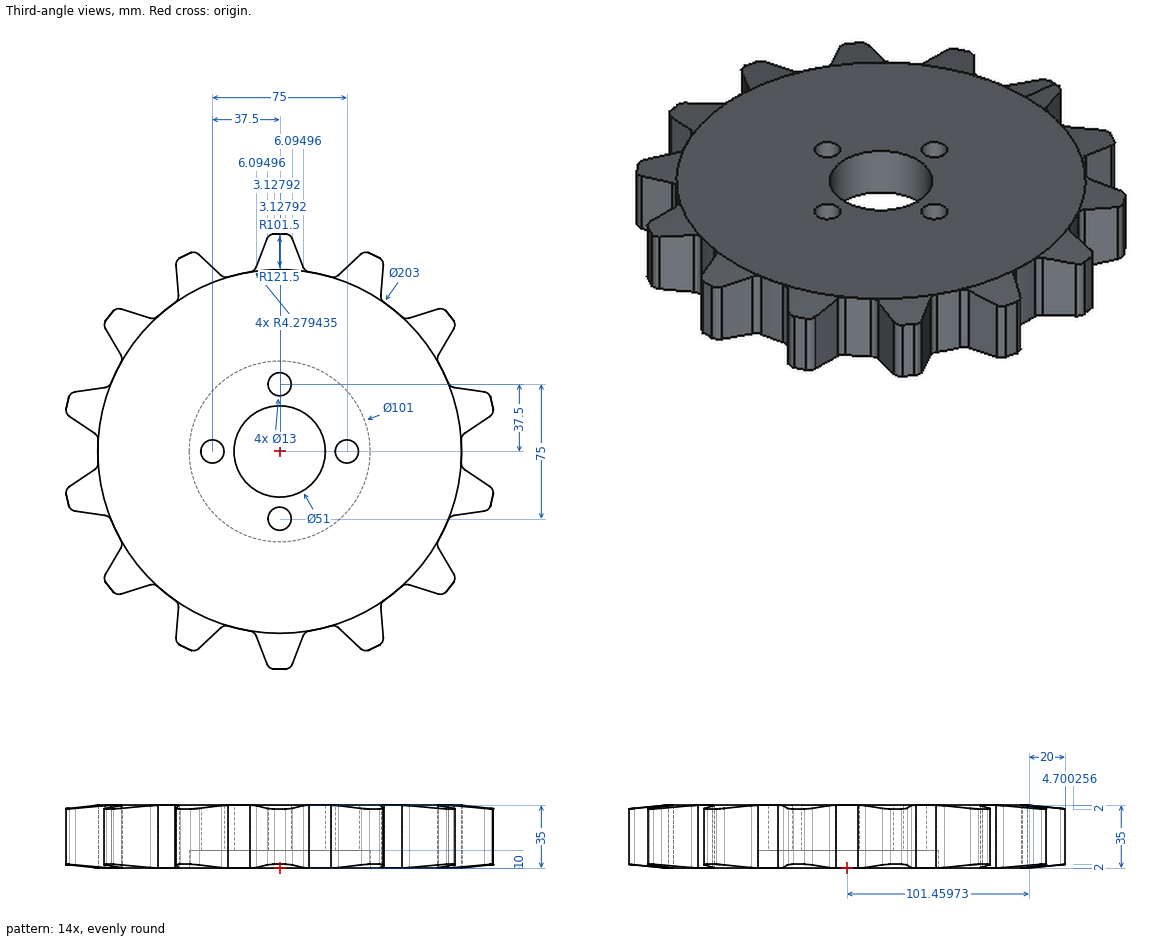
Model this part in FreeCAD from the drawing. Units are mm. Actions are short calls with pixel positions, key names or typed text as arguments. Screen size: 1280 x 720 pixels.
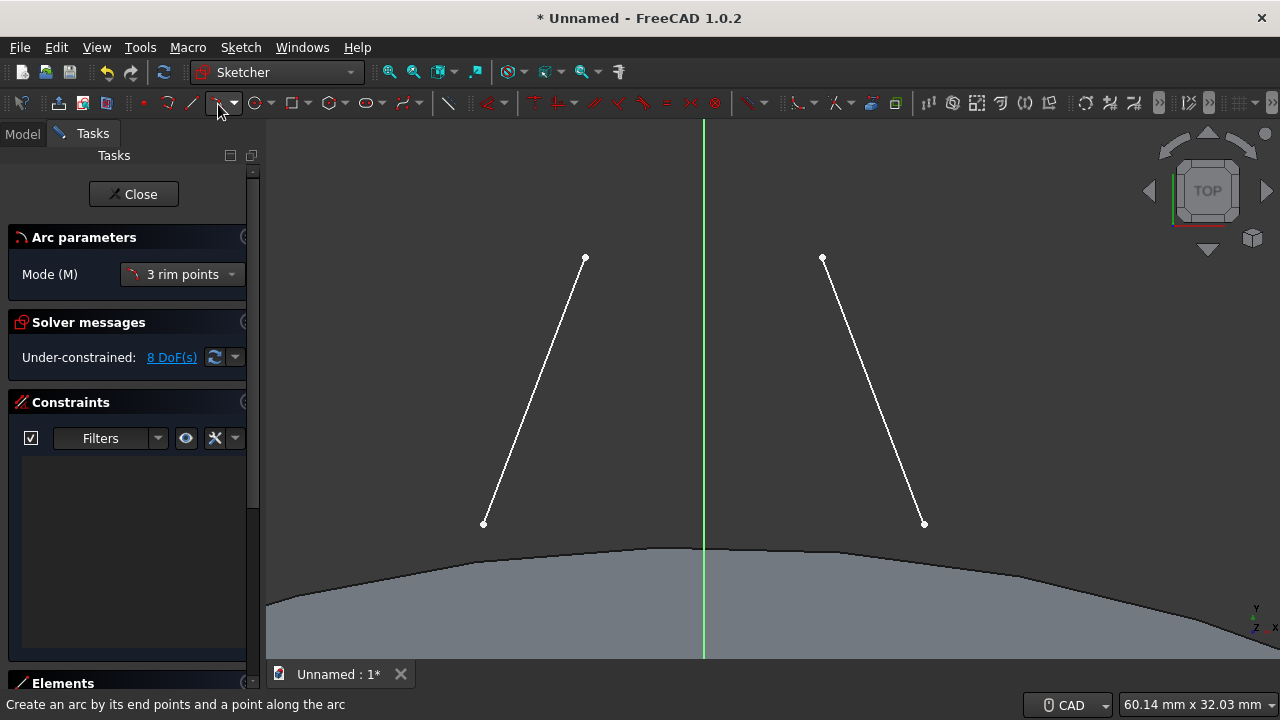
click(483, 525)
click(427, 570)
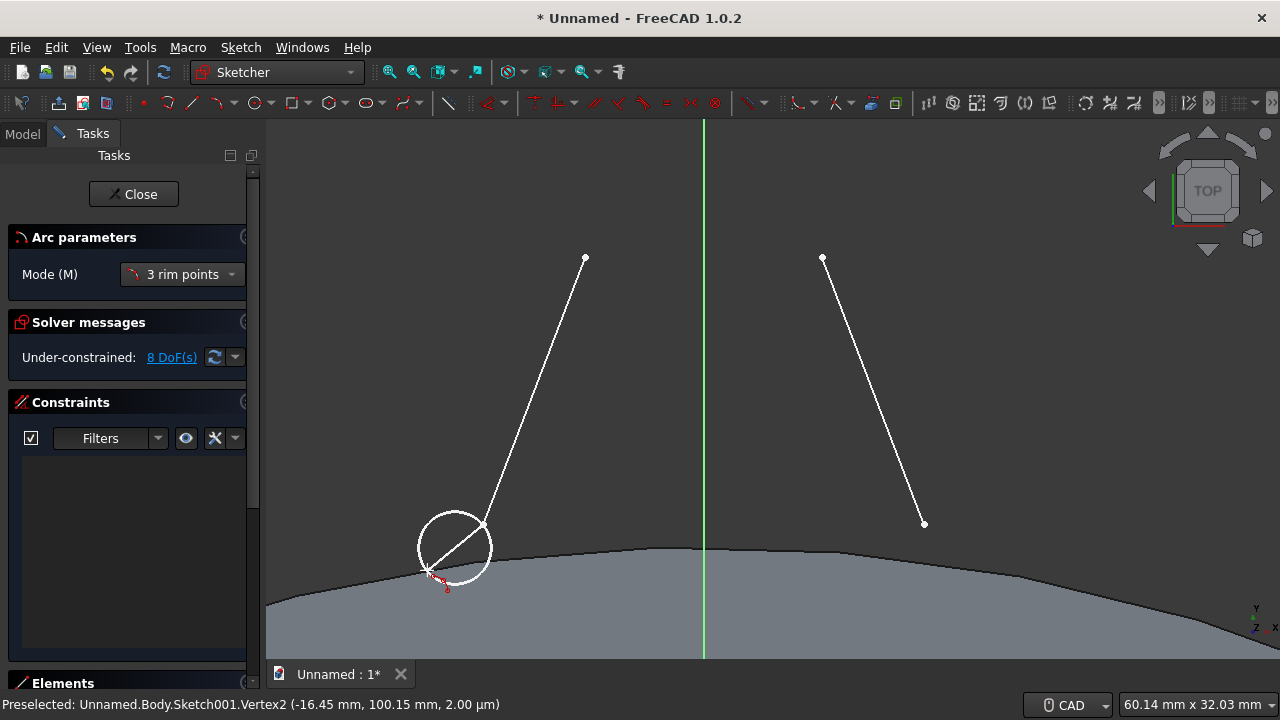
scroll(461, 554, up, 3)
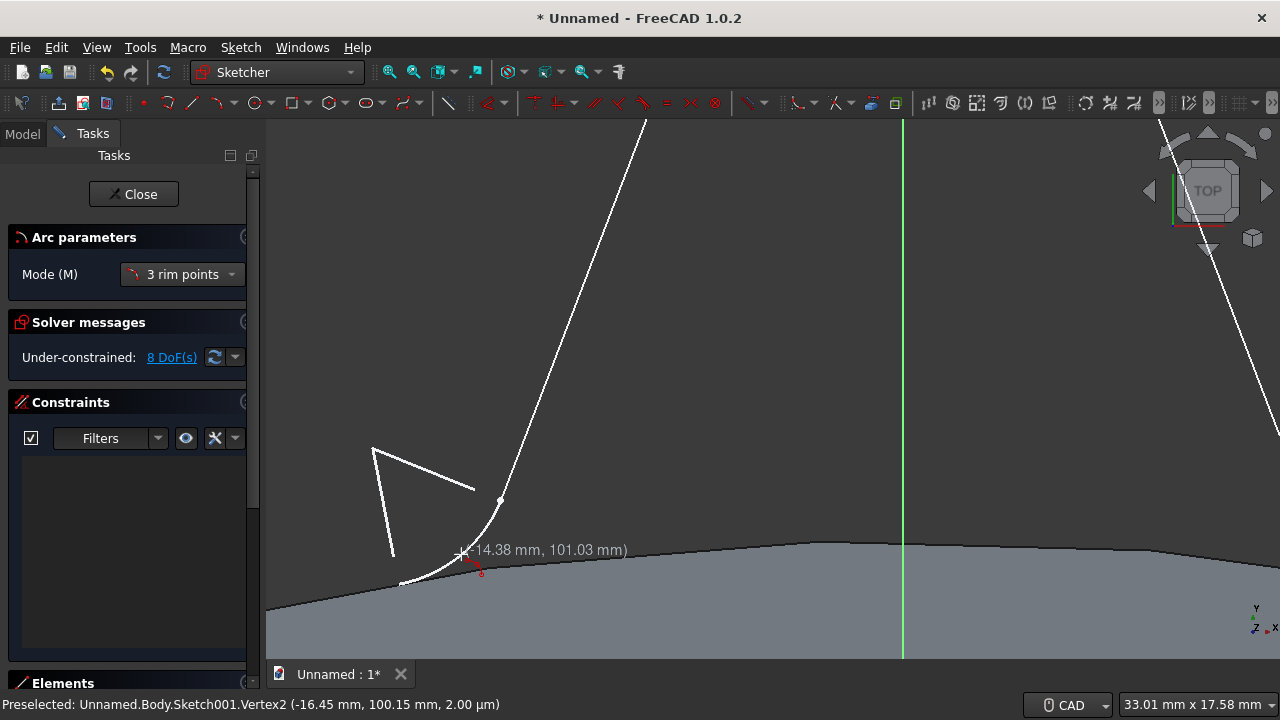
click(460, 554)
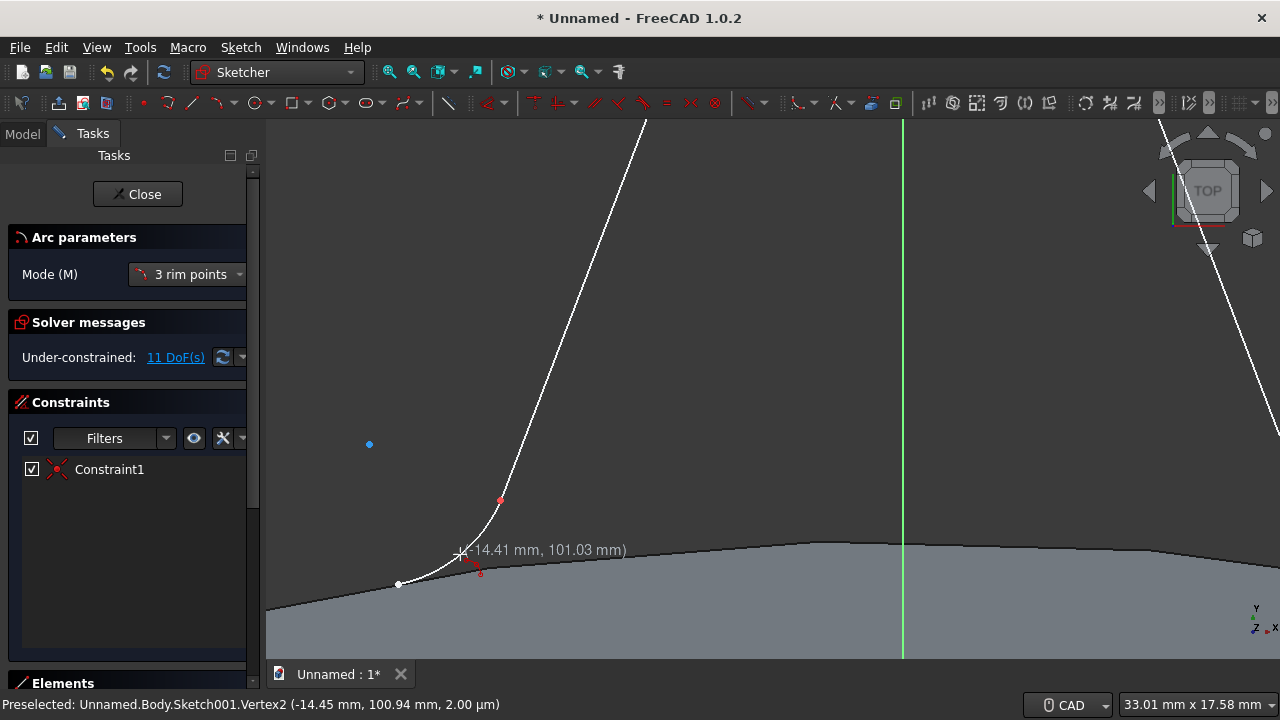
click(399, 584)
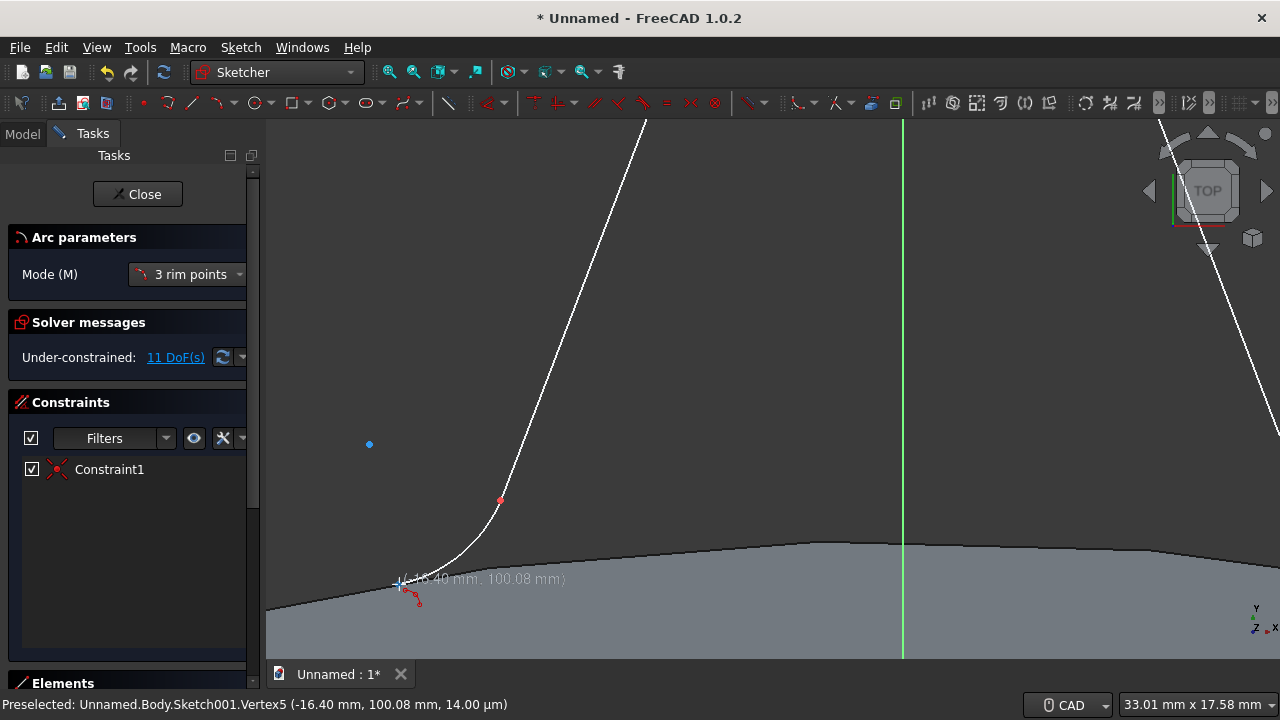
scroll(463, 553, down, 3)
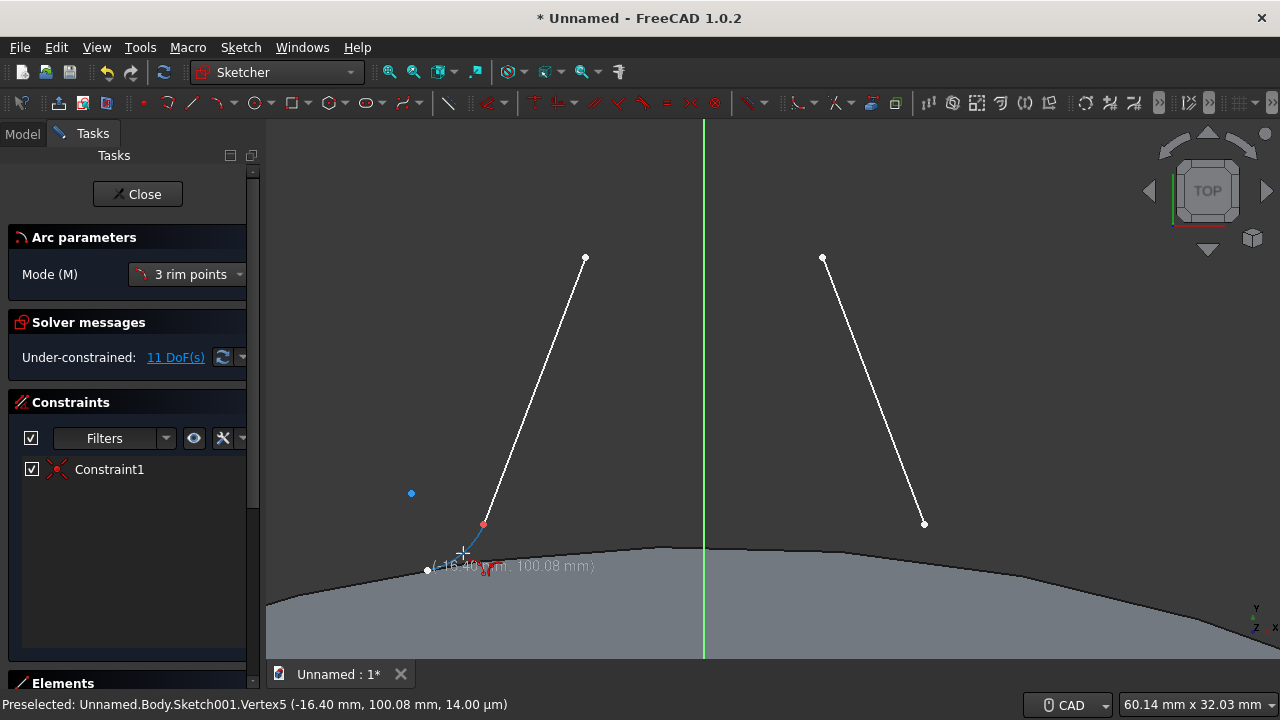
click(981, 569)
click(760, 547)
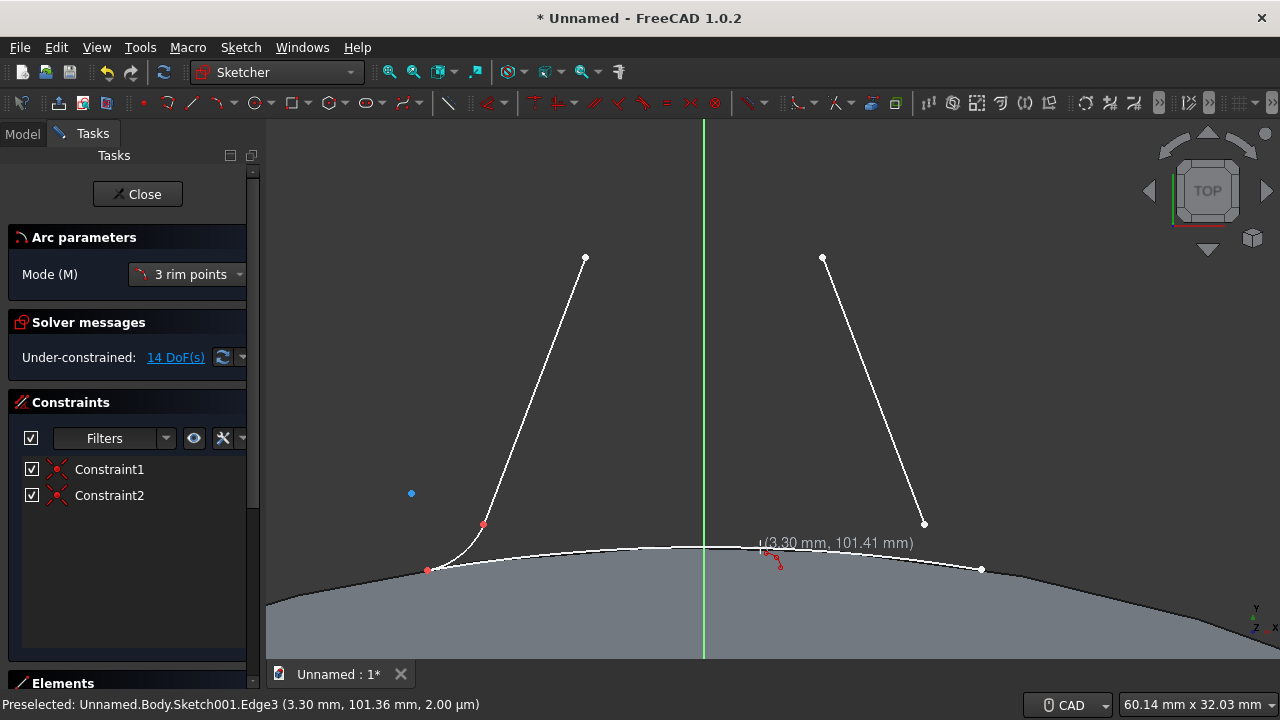
click(981, 570)
click(925, 525)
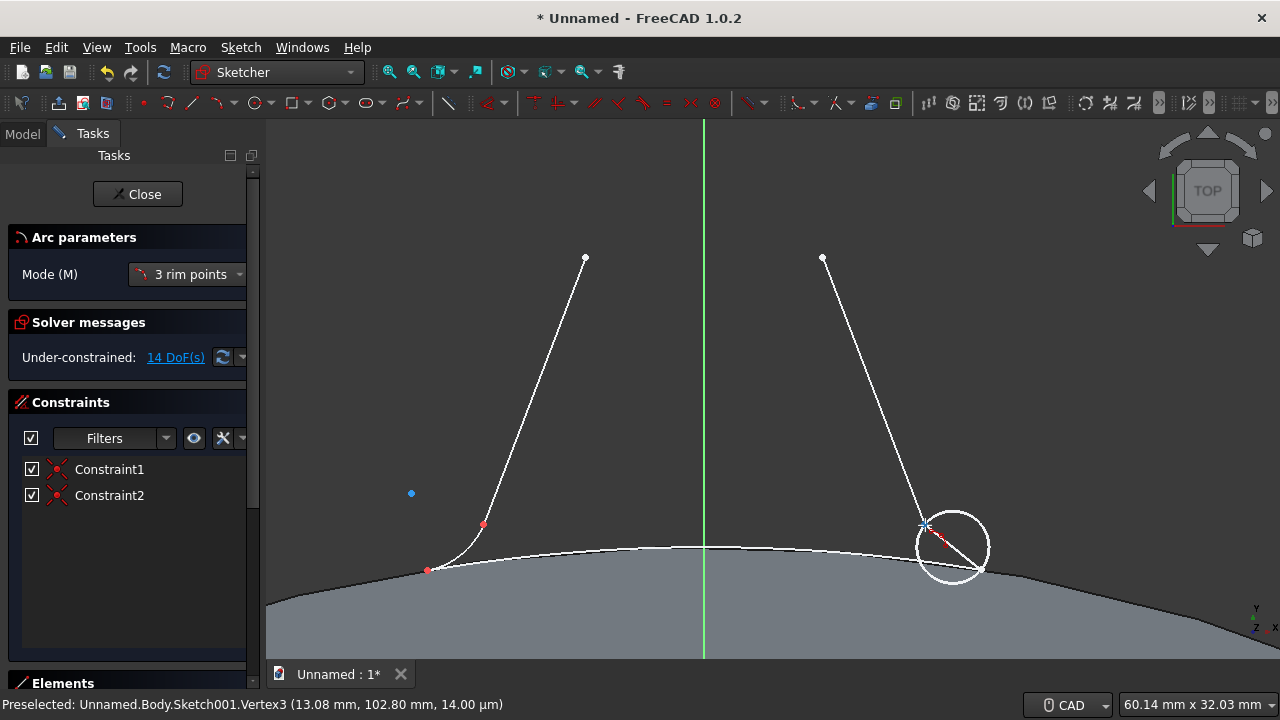
scroll(947, 554, up, 3)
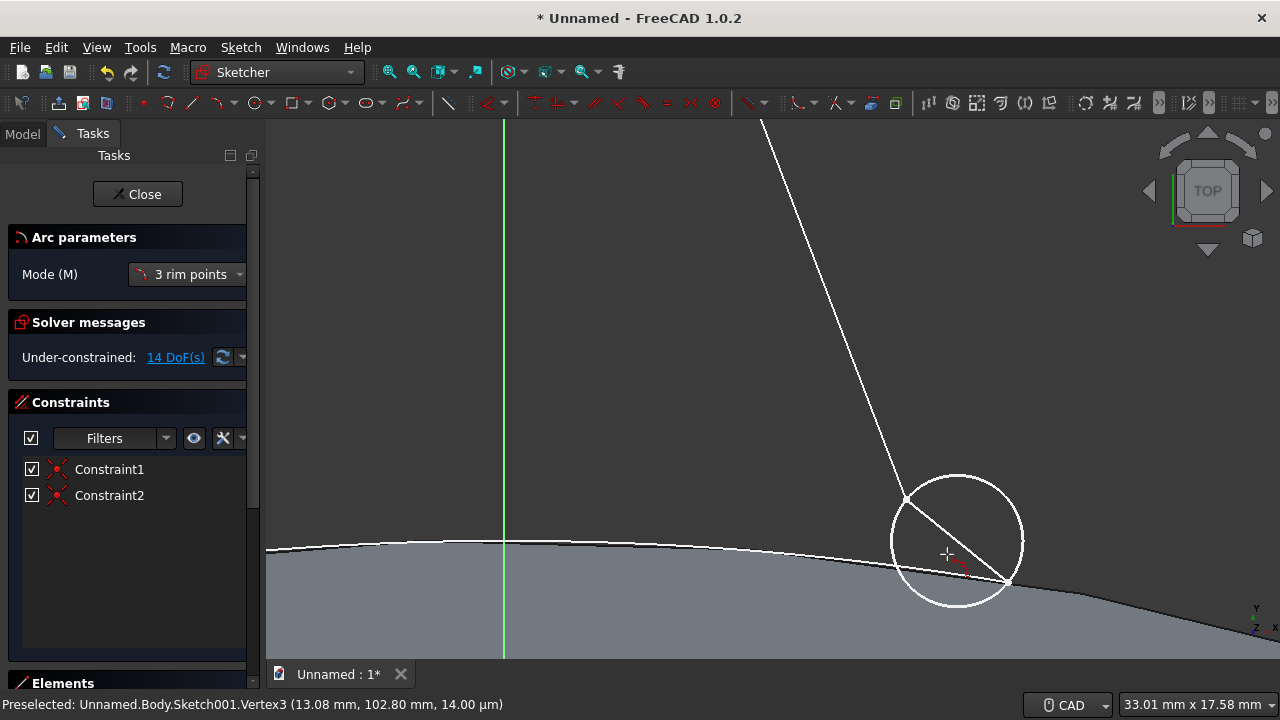
click(947, 553)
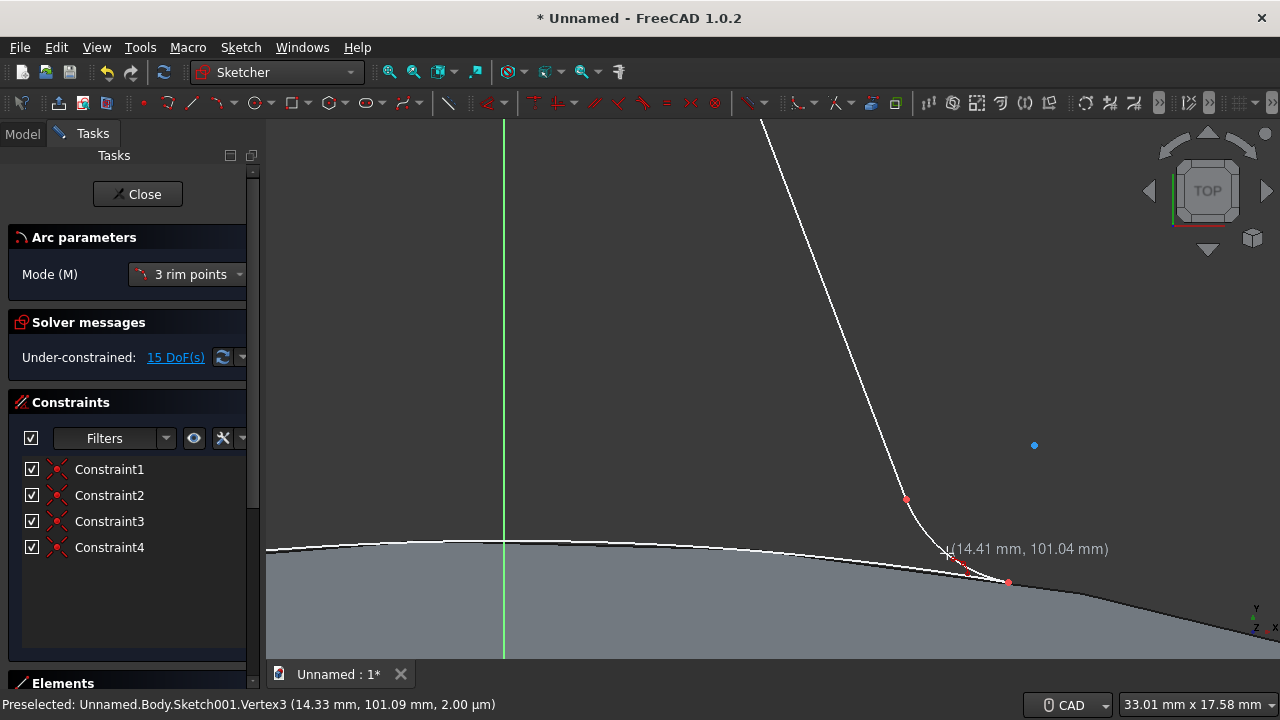
scroll(948, 554, down, 3)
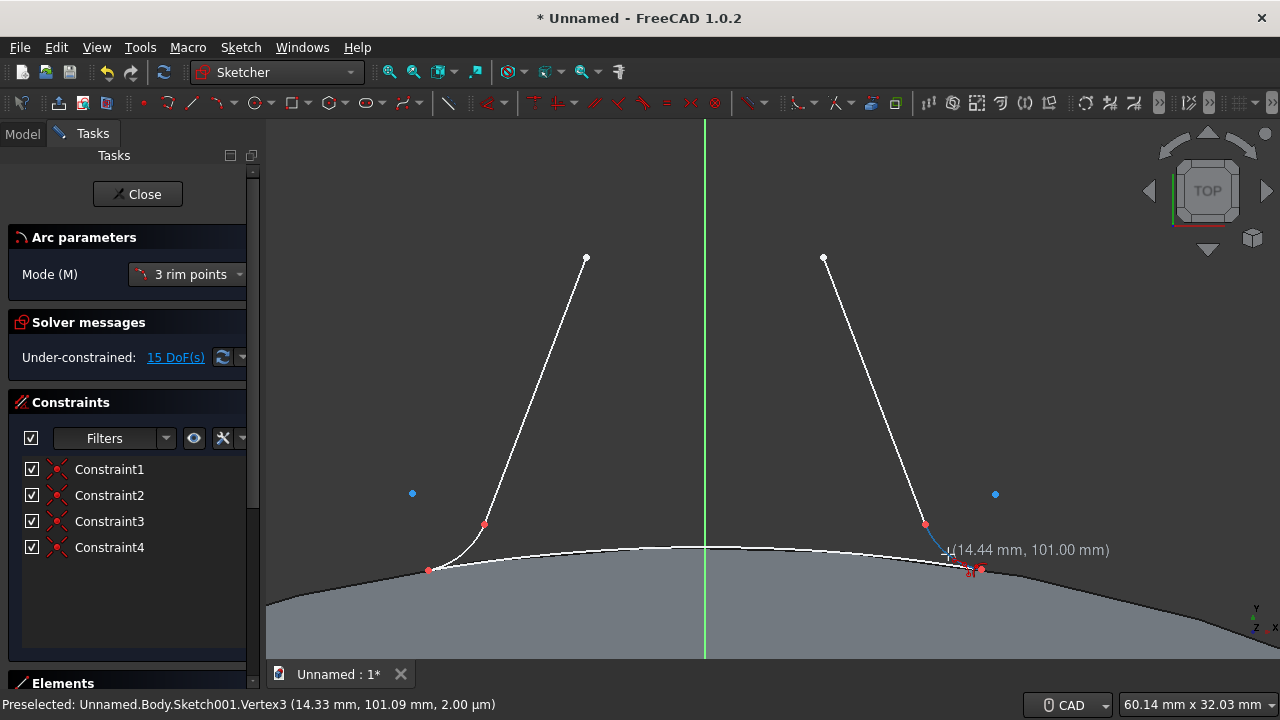
click(823, 258)
click(758, 210)